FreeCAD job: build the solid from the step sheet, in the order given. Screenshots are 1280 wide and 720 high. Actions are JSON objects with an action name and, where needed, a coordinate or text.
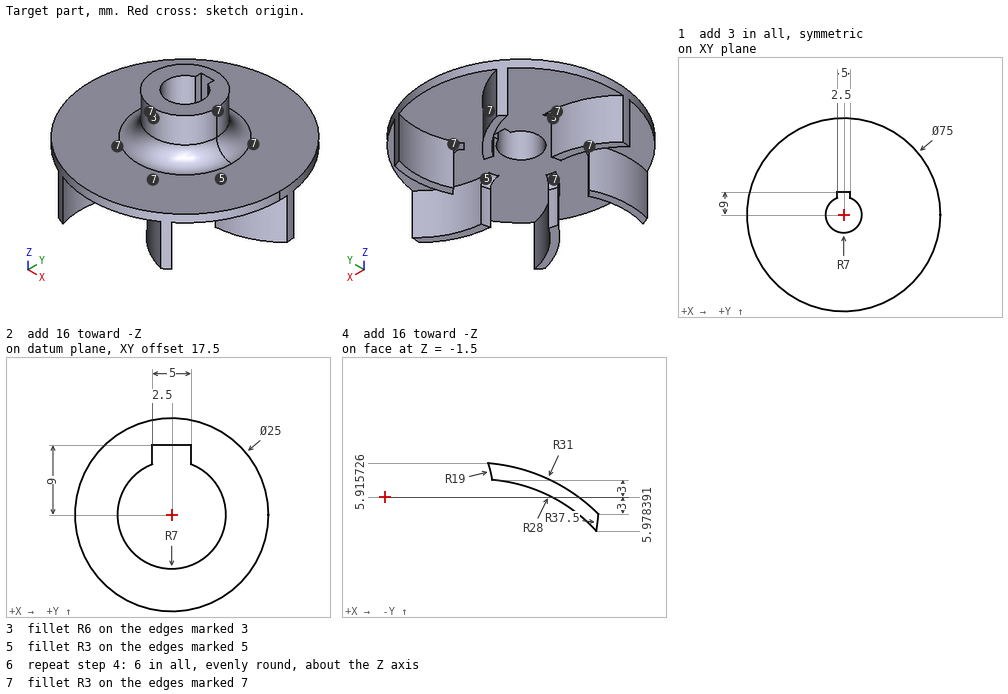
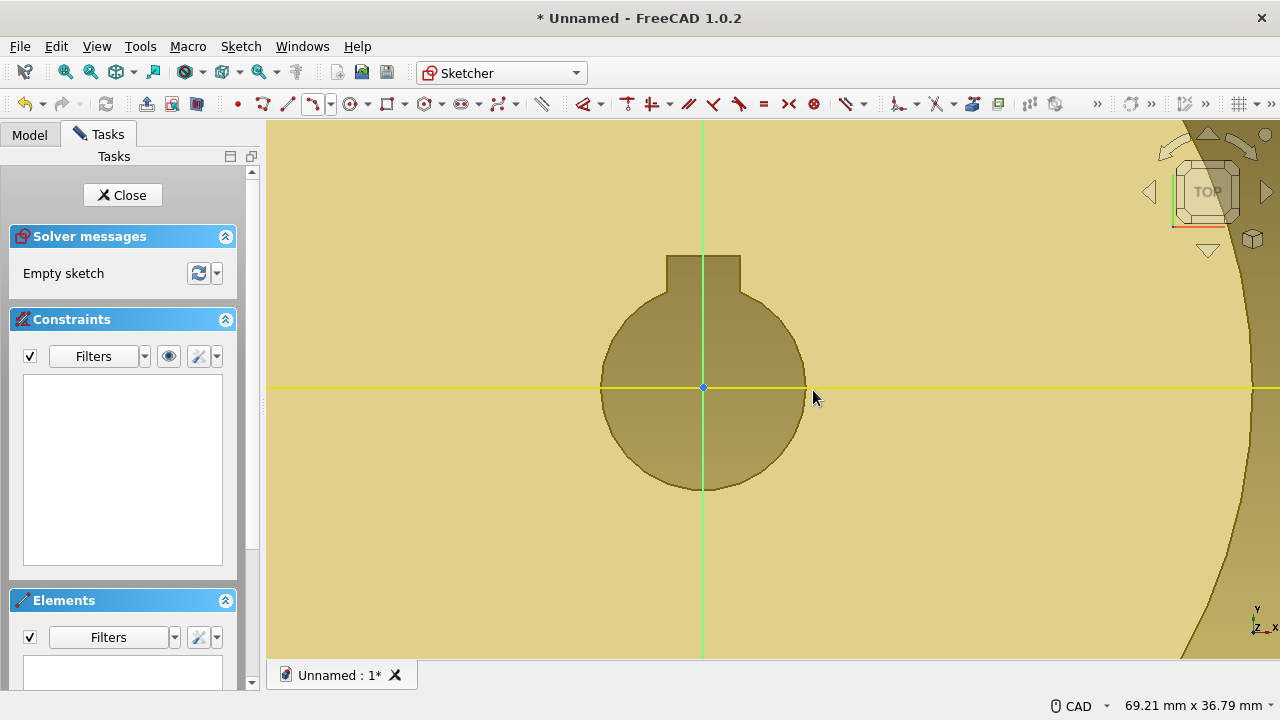
{"action": "key", "text": "g m"}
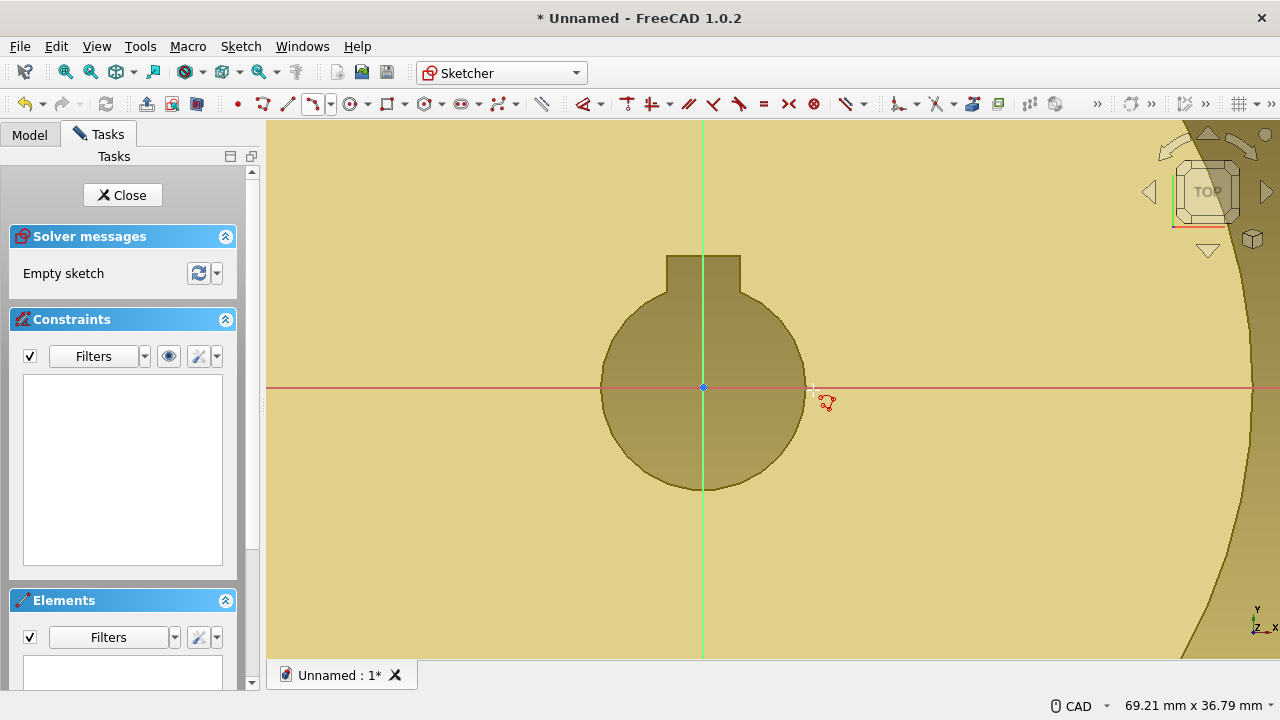
{"action": "left_click", "coordinate": [667, 292]}
{"action": "left_click", "coordinate": [667, 256]}
{"action": "left_click", "coordinate": [740, 256]}
{"action": "left_click", "coordinate": [740, 292]}
{"action": "right_click", "coordinate": [740, 292]}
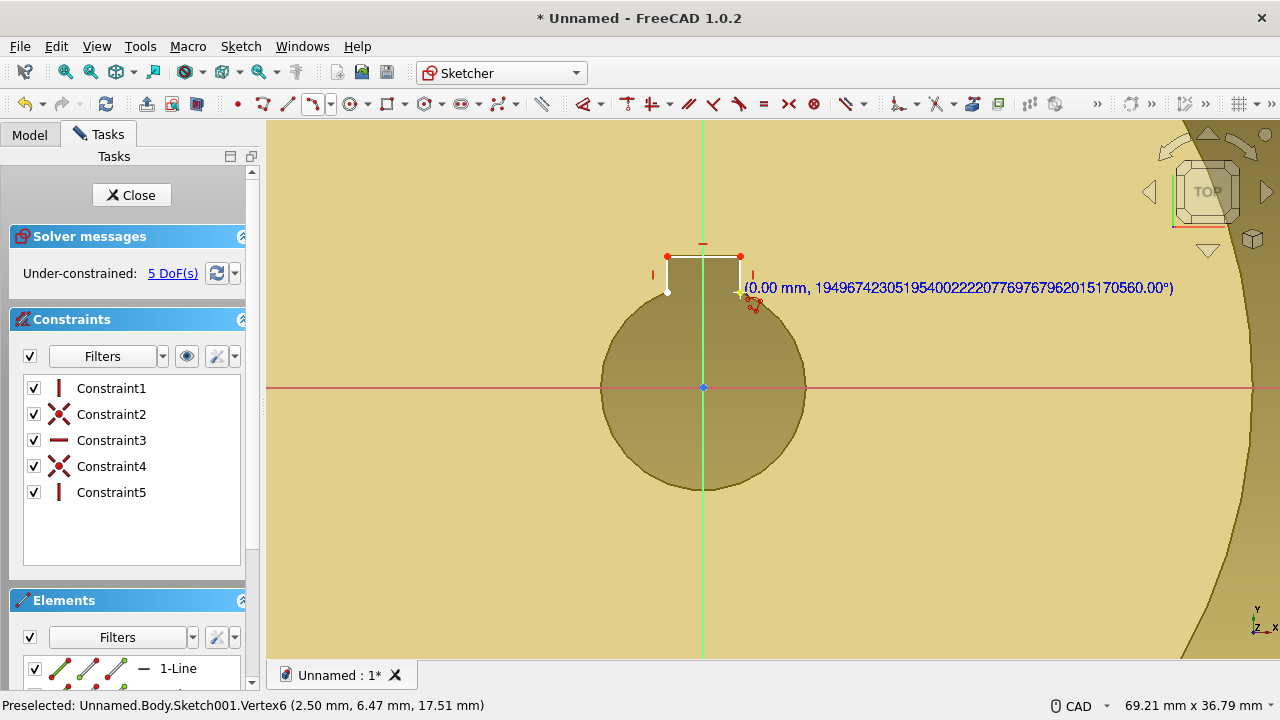
{"action": "left_click", "coordinate": [312, 104]}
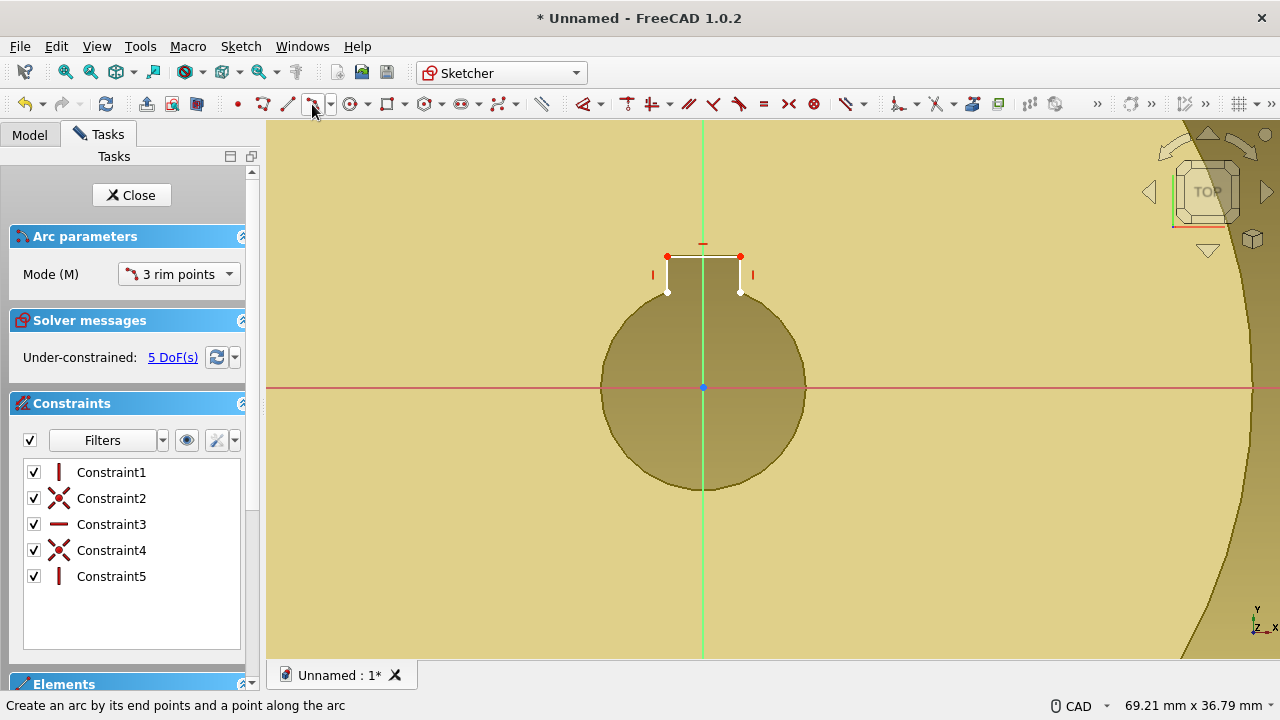
{"action": "left_click", "coordinate": [740, 293]}
{"action": "left_click", "coordinate": [667, 293]}
{"action": "left_click", "coordinate": [649, 475]}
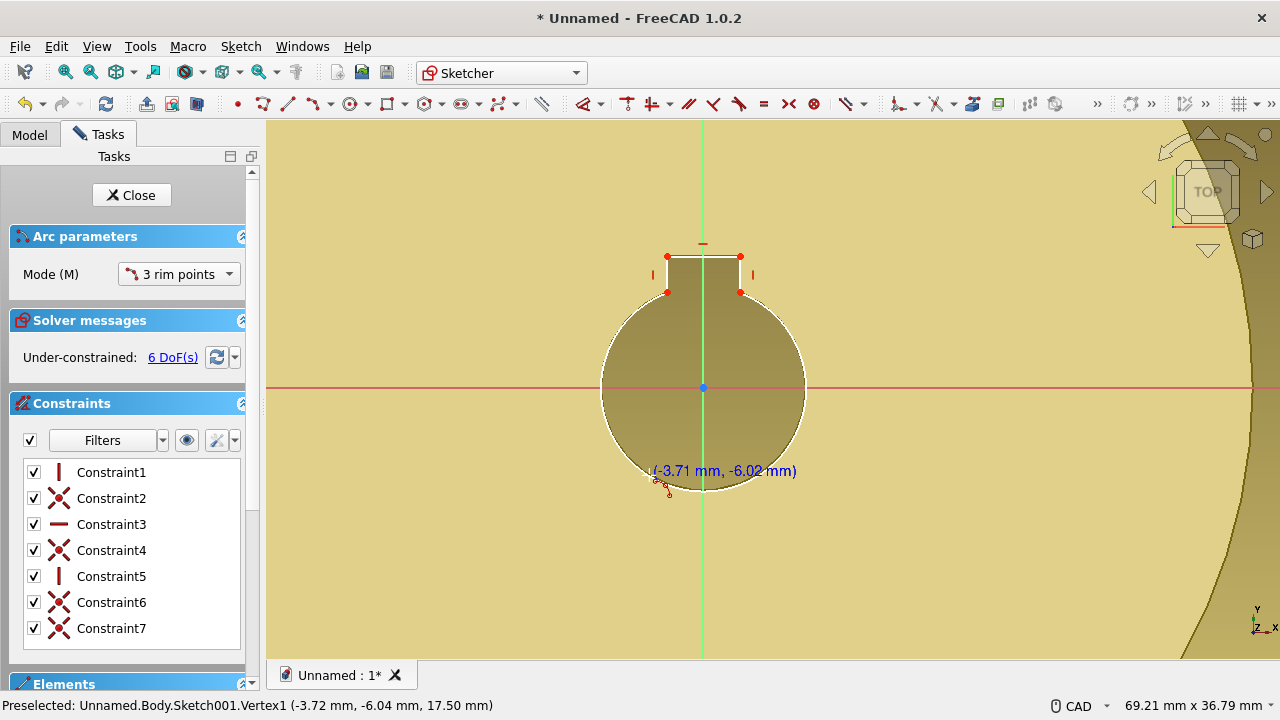
{"action": "left_click", "coordinate": [350, 104]}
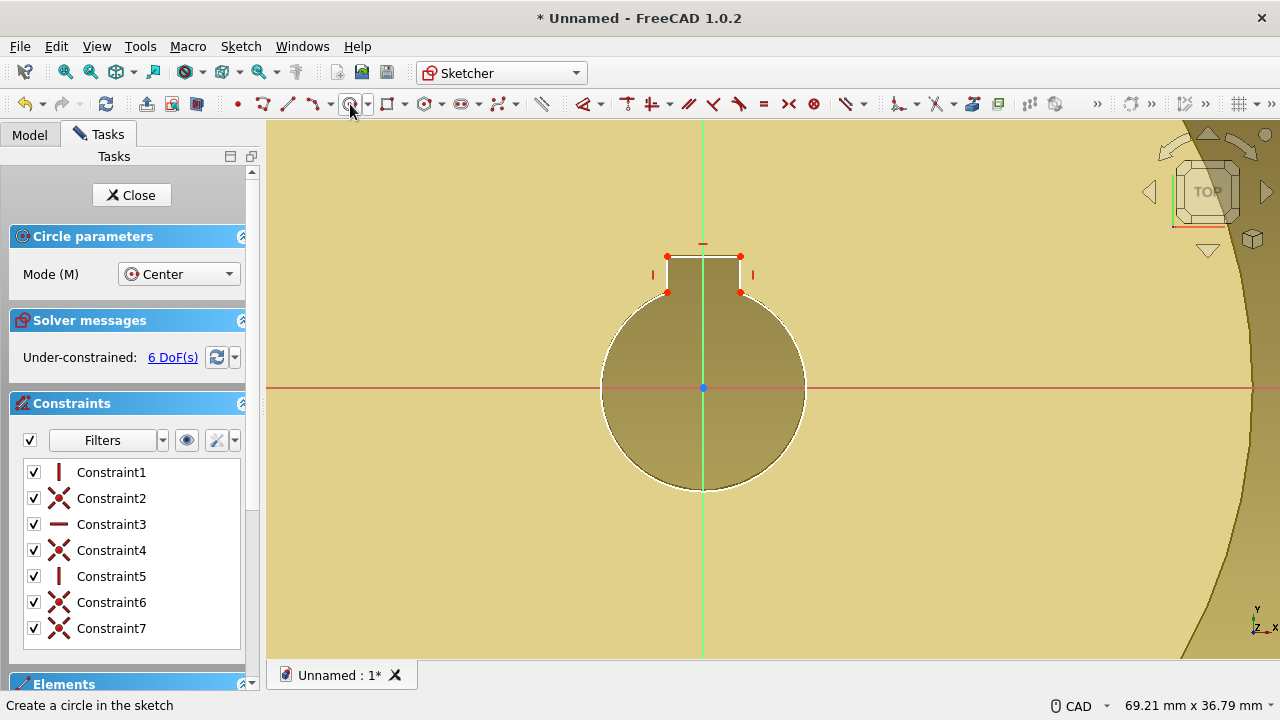
{"action": "left_click", "coordinate": [703, 388]}
{"action": "mouse_move", "coordinate": [833, 258]}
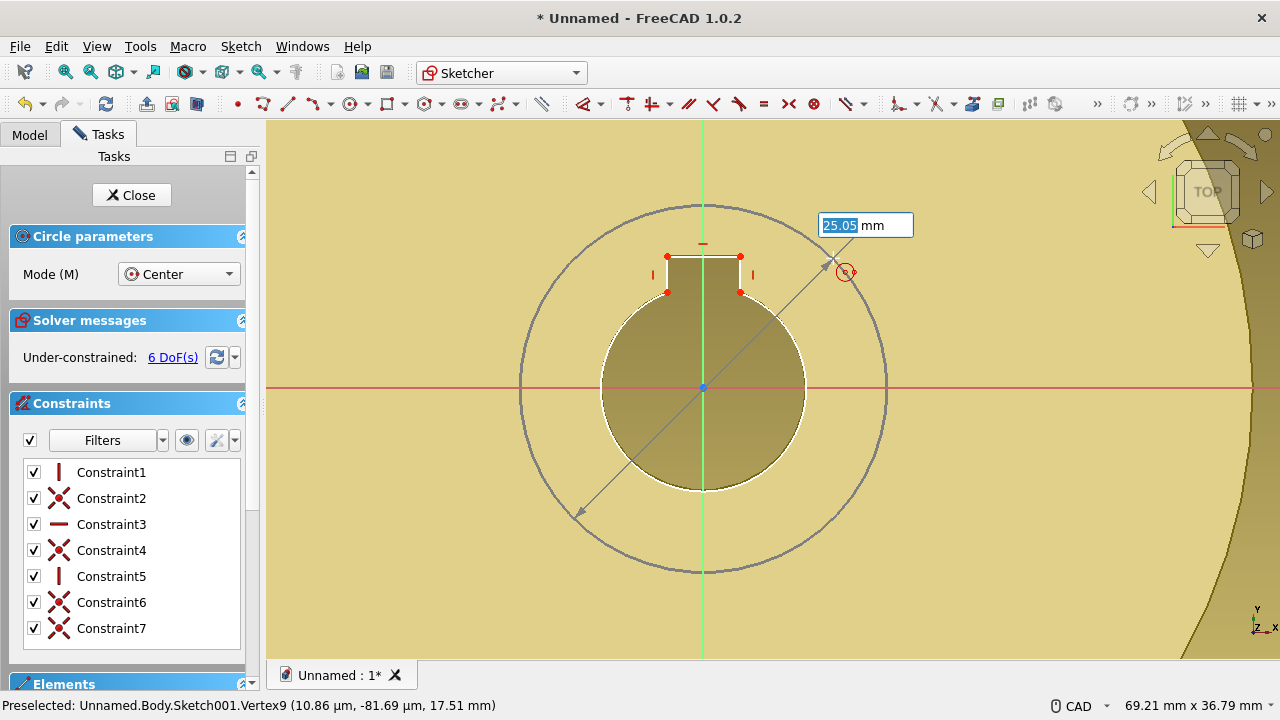
{"action": "type", "text": "25"}
{"action": "key", "text": "Return"}
{"action": "key", "text": "Escape"}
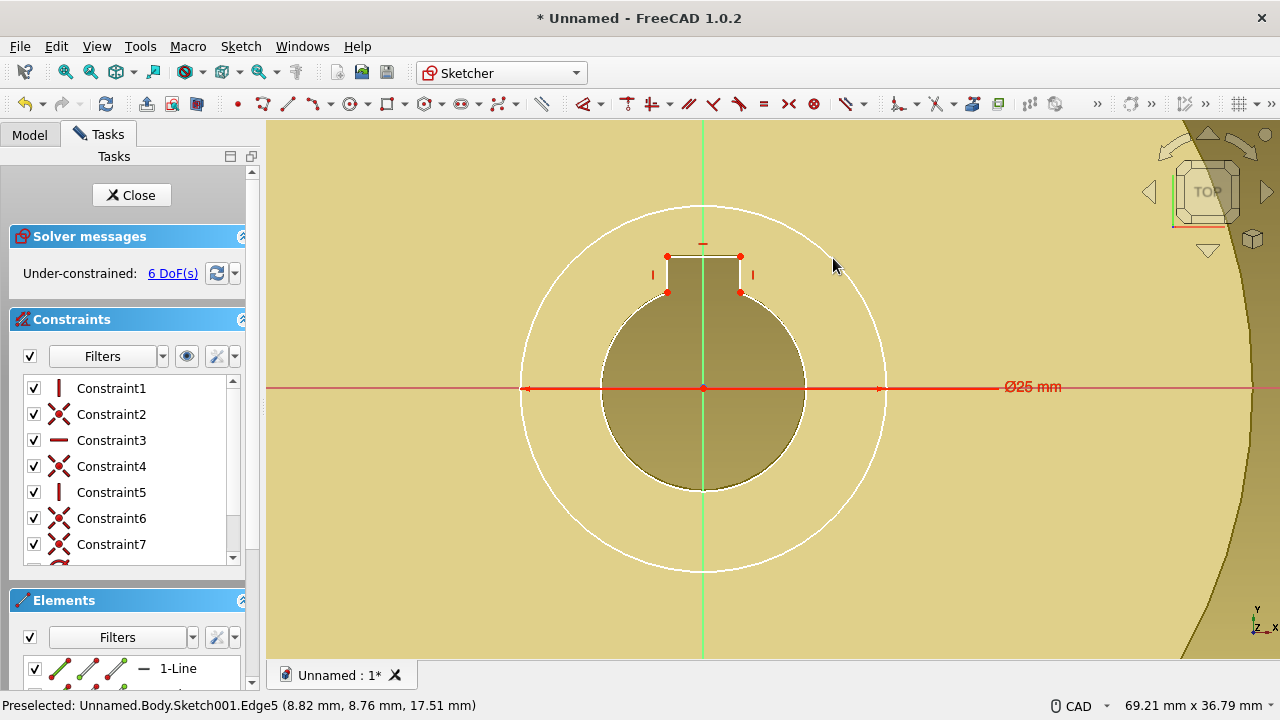
{"action": "left_click_drag", "start_coordinate": [693, 378], "coordinate": [713, 399]}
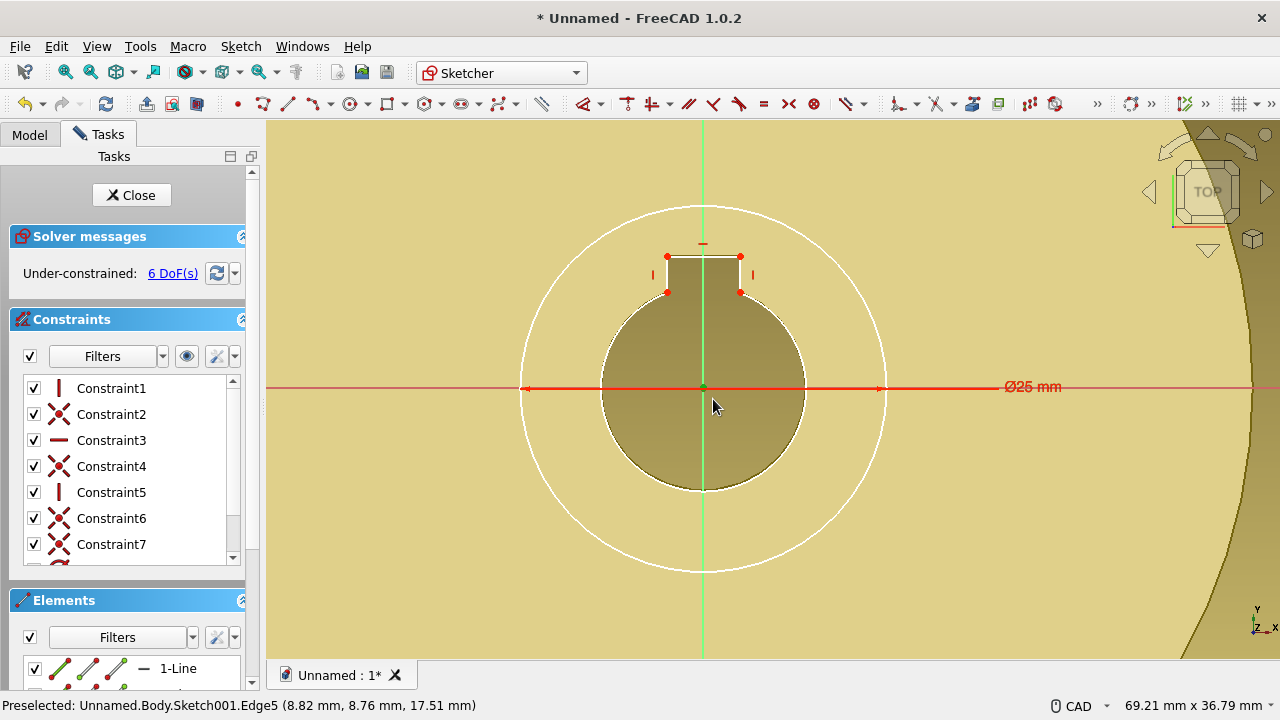
{"action": "left_click", "coordinate": [627, 104]}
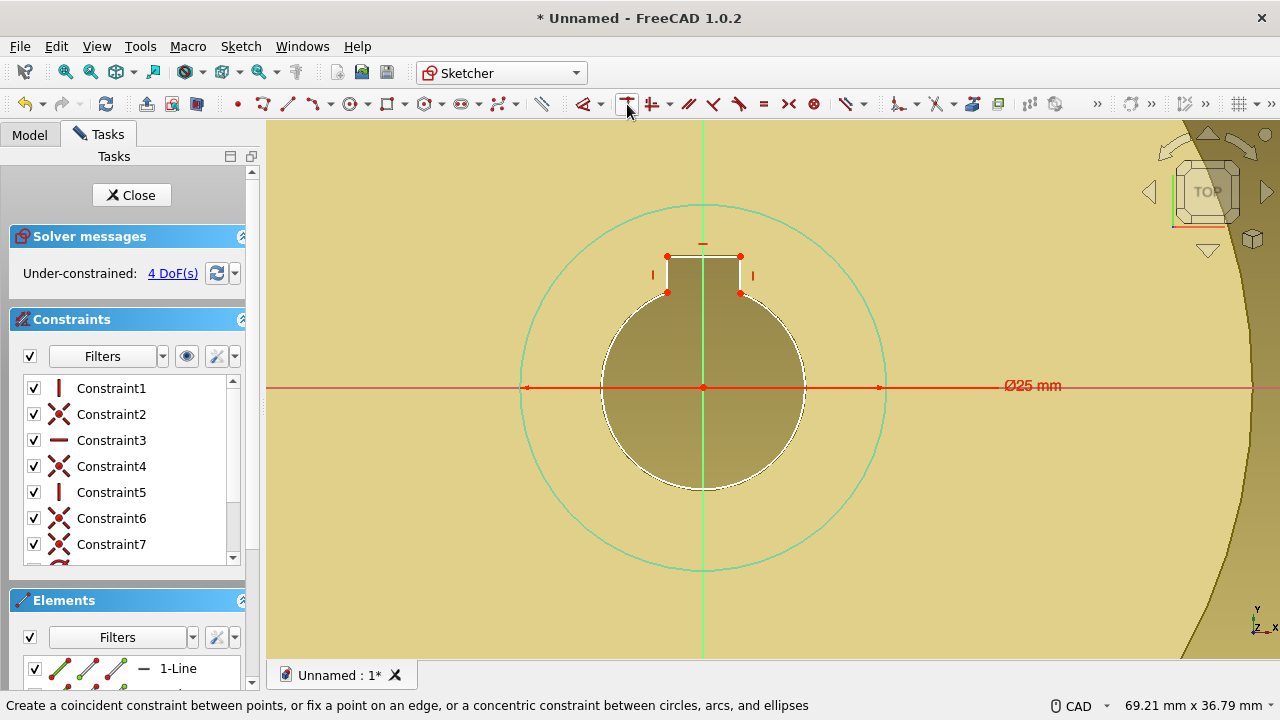
{"action": "left_click", "coordinate": [582, 104]}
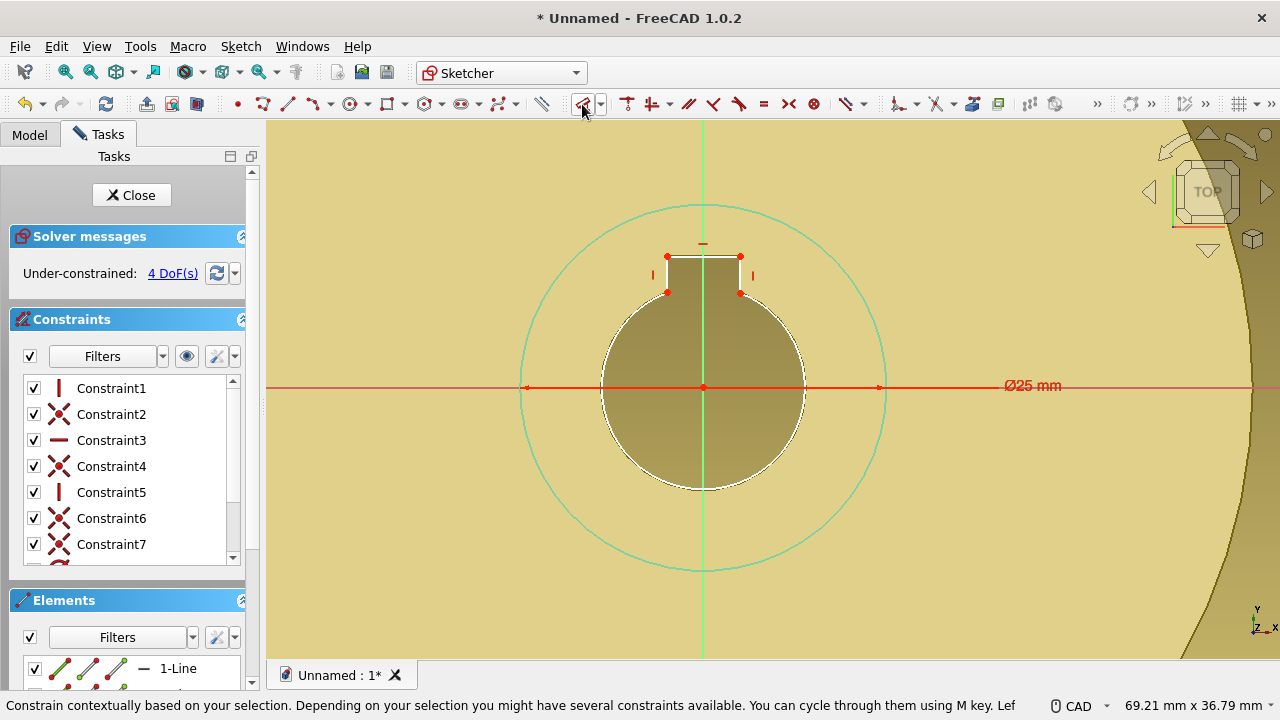
{"action": "left_click", "coordinate": [612, 433]}
{"action": "left_click", "coordinate": [583, 447]}